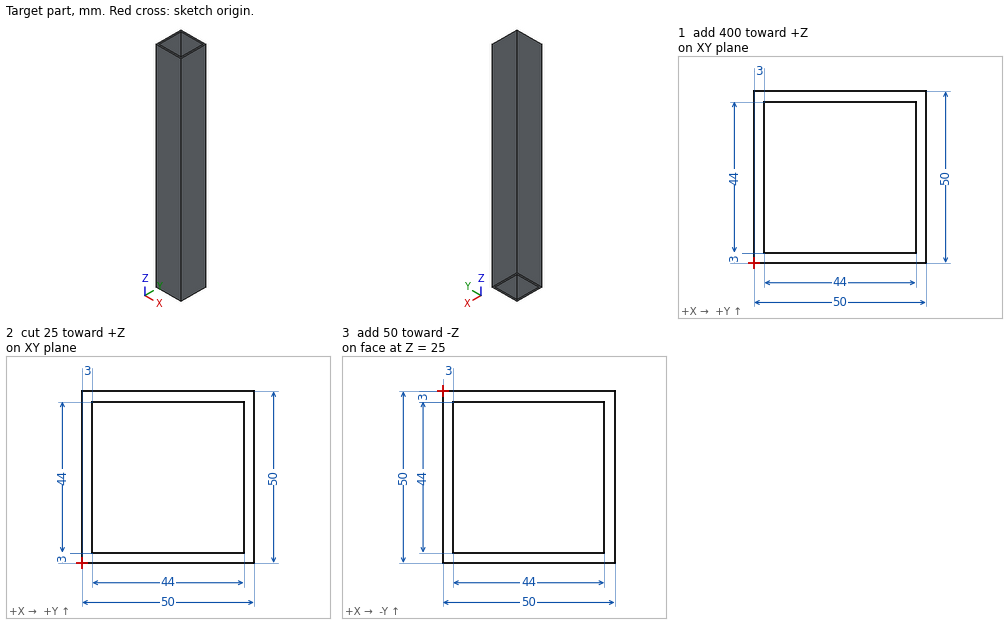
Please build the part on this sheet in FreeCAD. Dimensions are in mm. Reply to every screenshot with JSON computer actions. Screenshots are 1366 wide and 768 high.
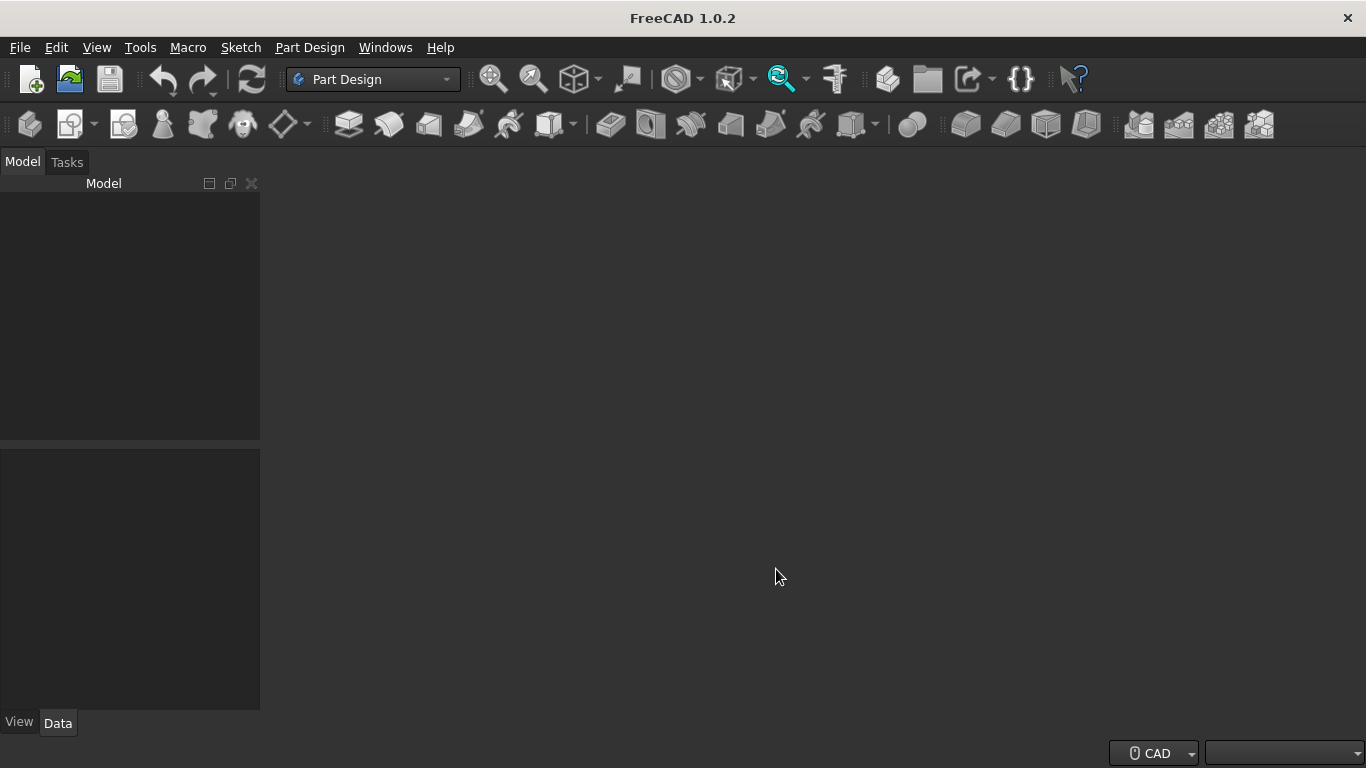
{"action": "left_click", "coordinate": [30, 80]}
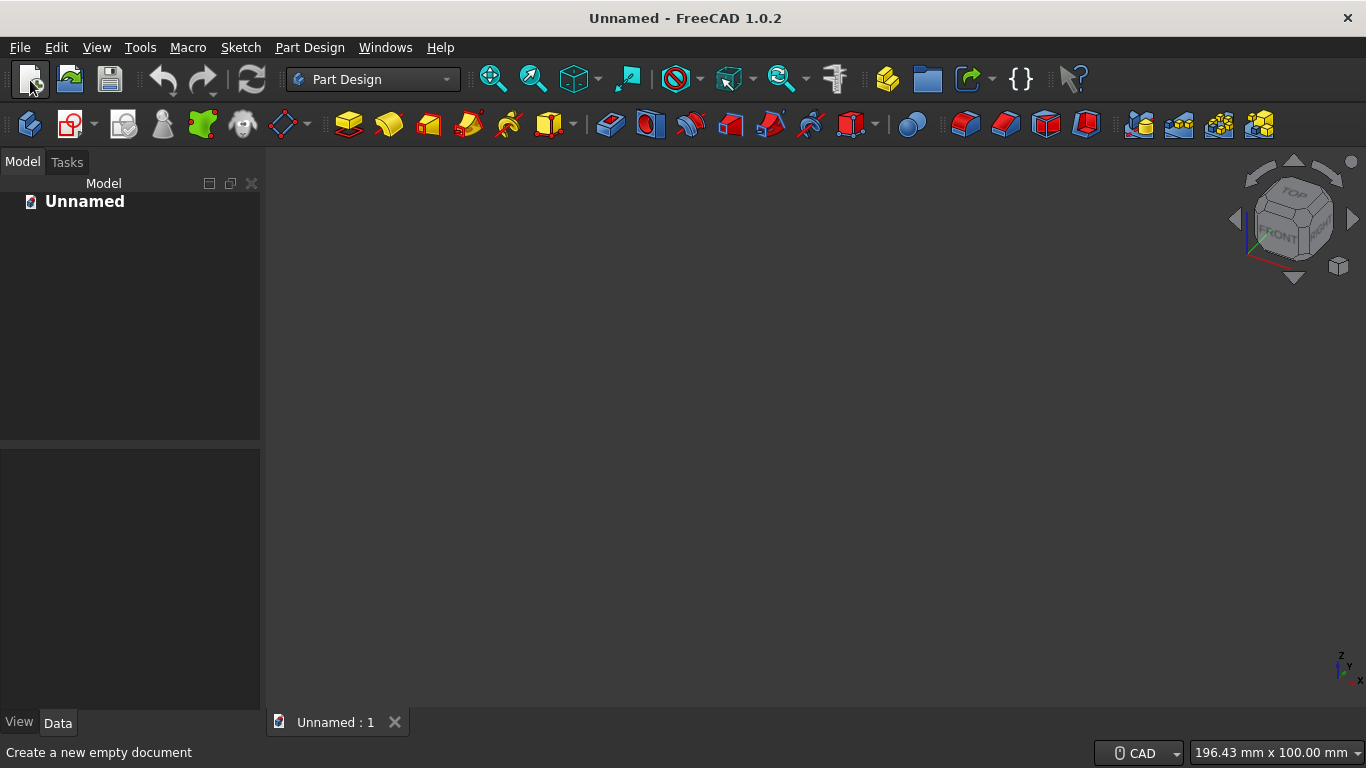
{"action": "left_click", "coordinate": [70, 124]}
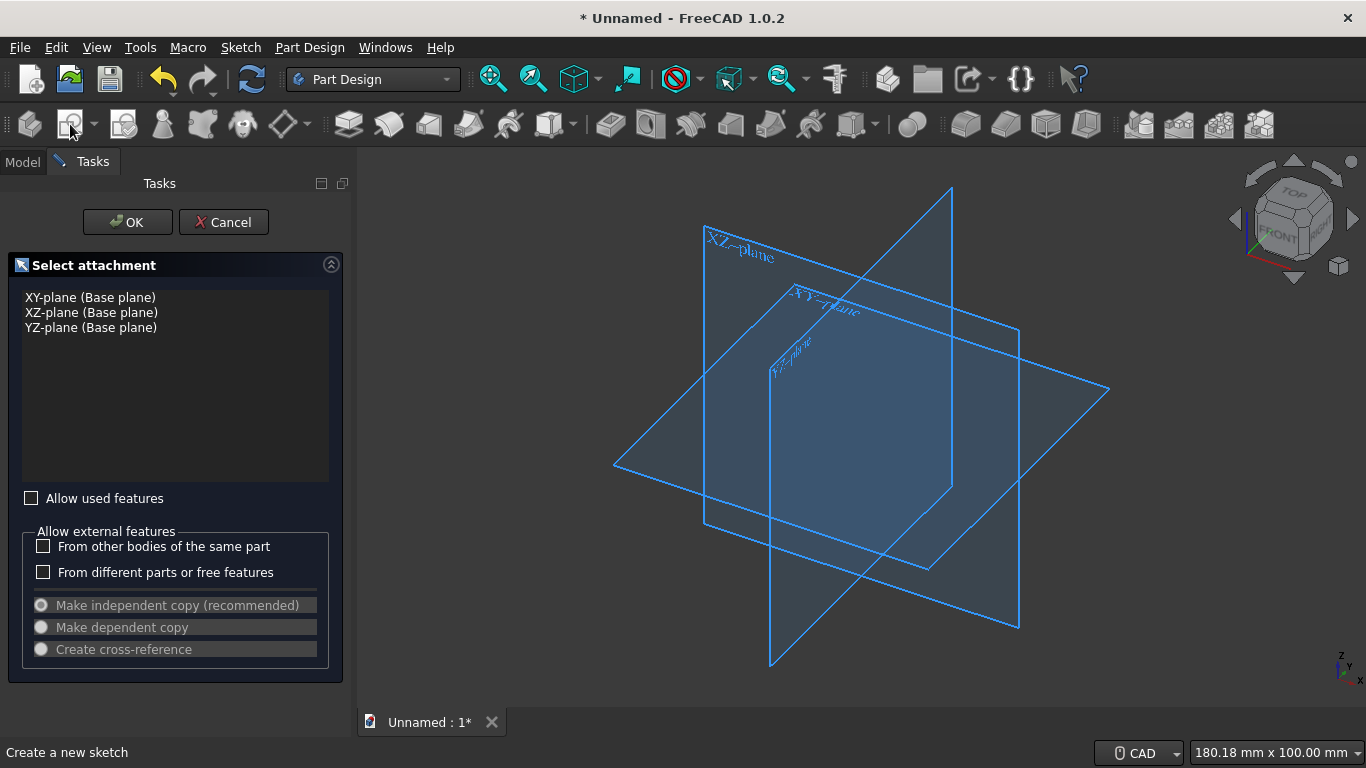
{"action": "left_click", "coordinate": [82, 298]}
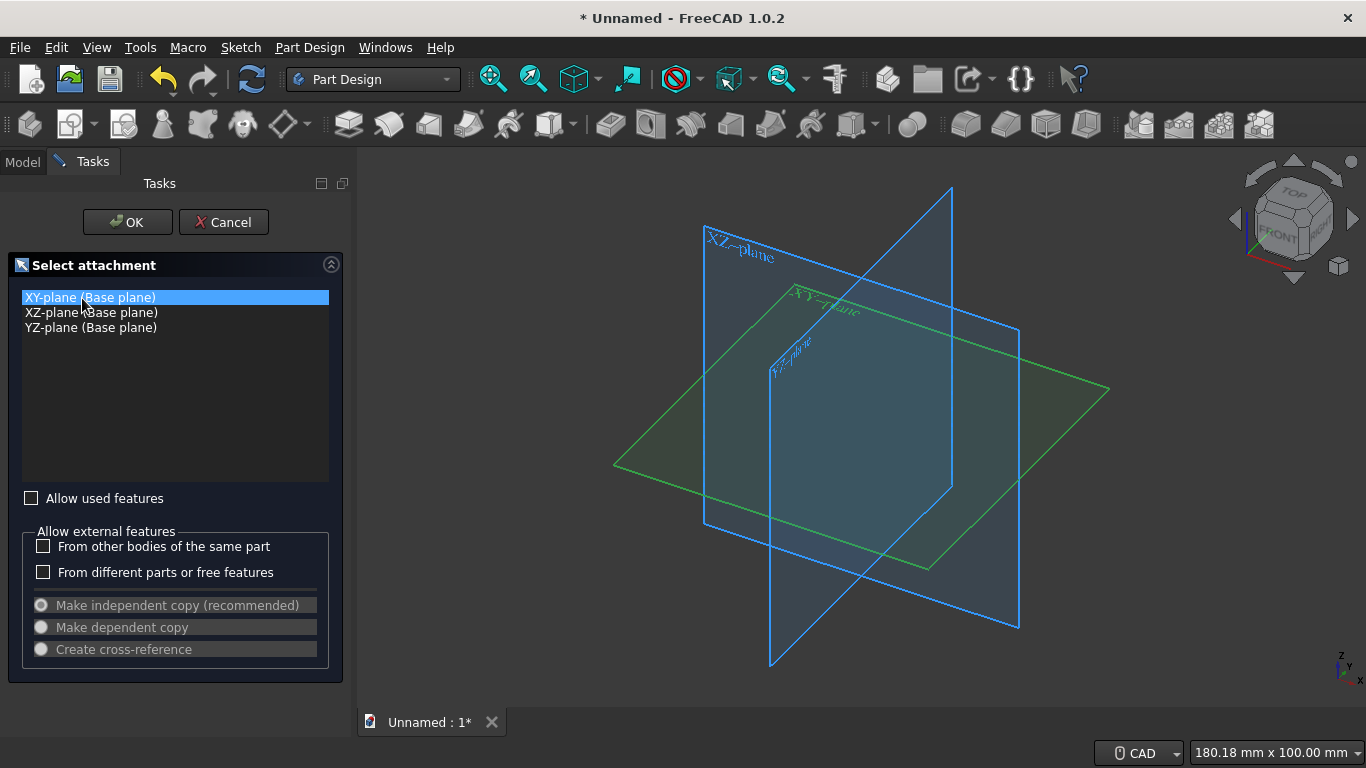
{"action": "left_click", "coordinate": [128, 222]}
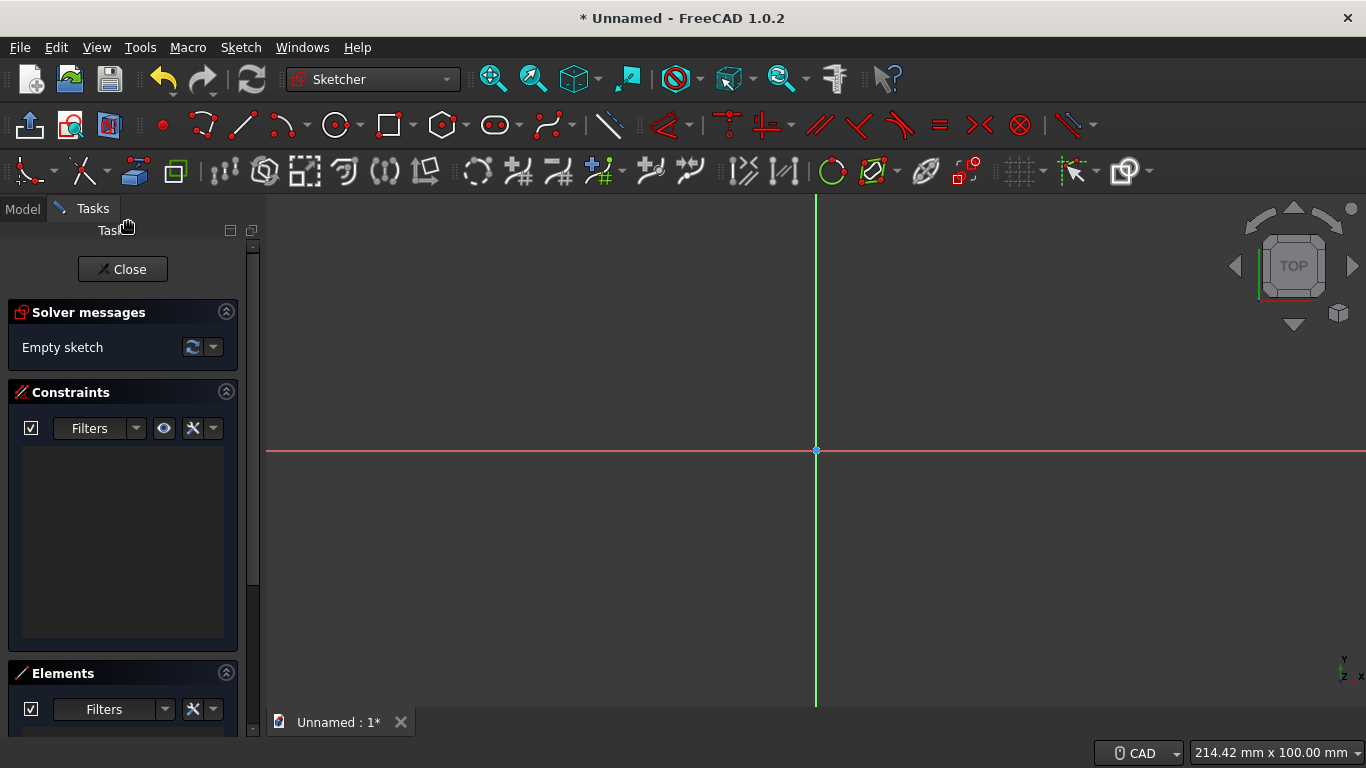
{"action": "scroll", "coordinate": [294, 679], "scroll_direction": "down", "scroll_amount": 1}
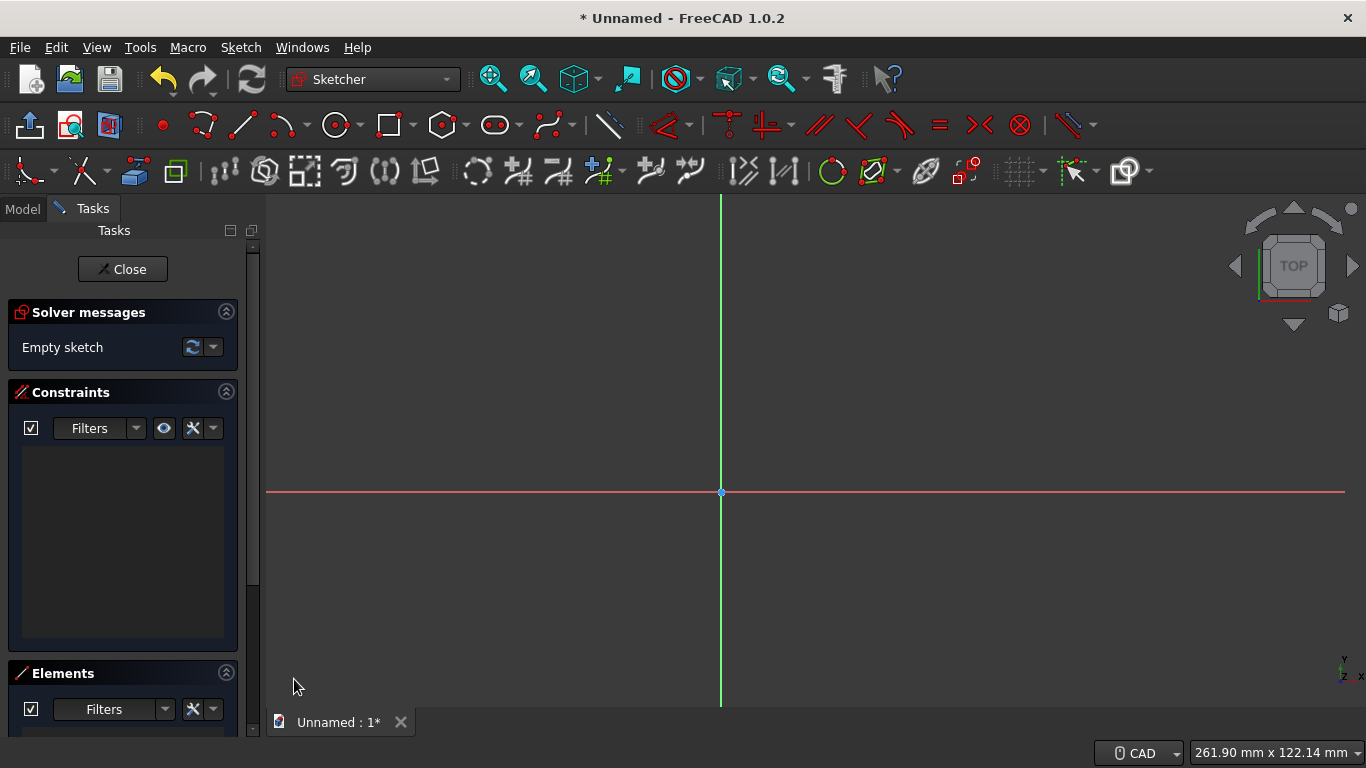
{"action": "scroll", "coordinate": [987, 258], "scroll_direction": "up", "scroll_amount": 2}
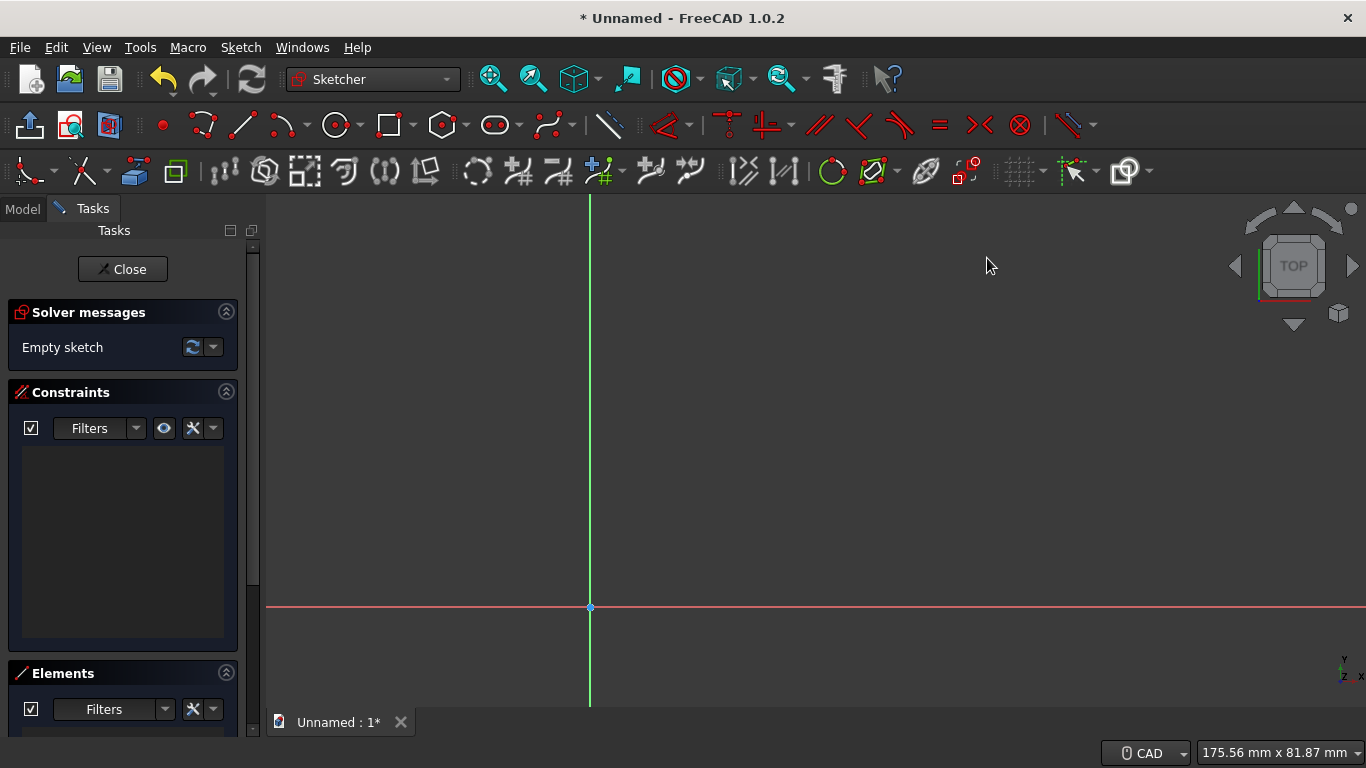
{"action": "left_click", "coordinate": [390, 126]}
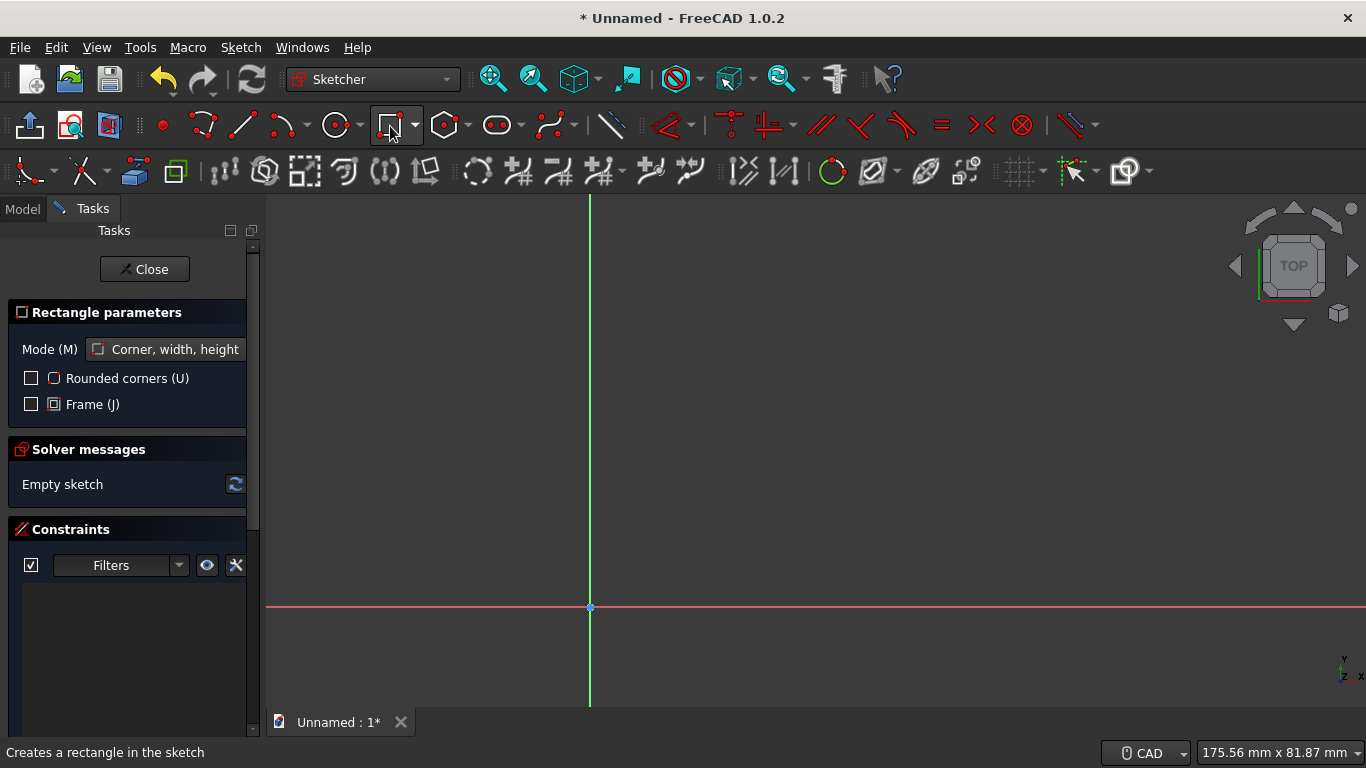
{"action": "left_click", "coordinate": [590, 607]}
{"action": "left_click", "coordinate": [904, 294]}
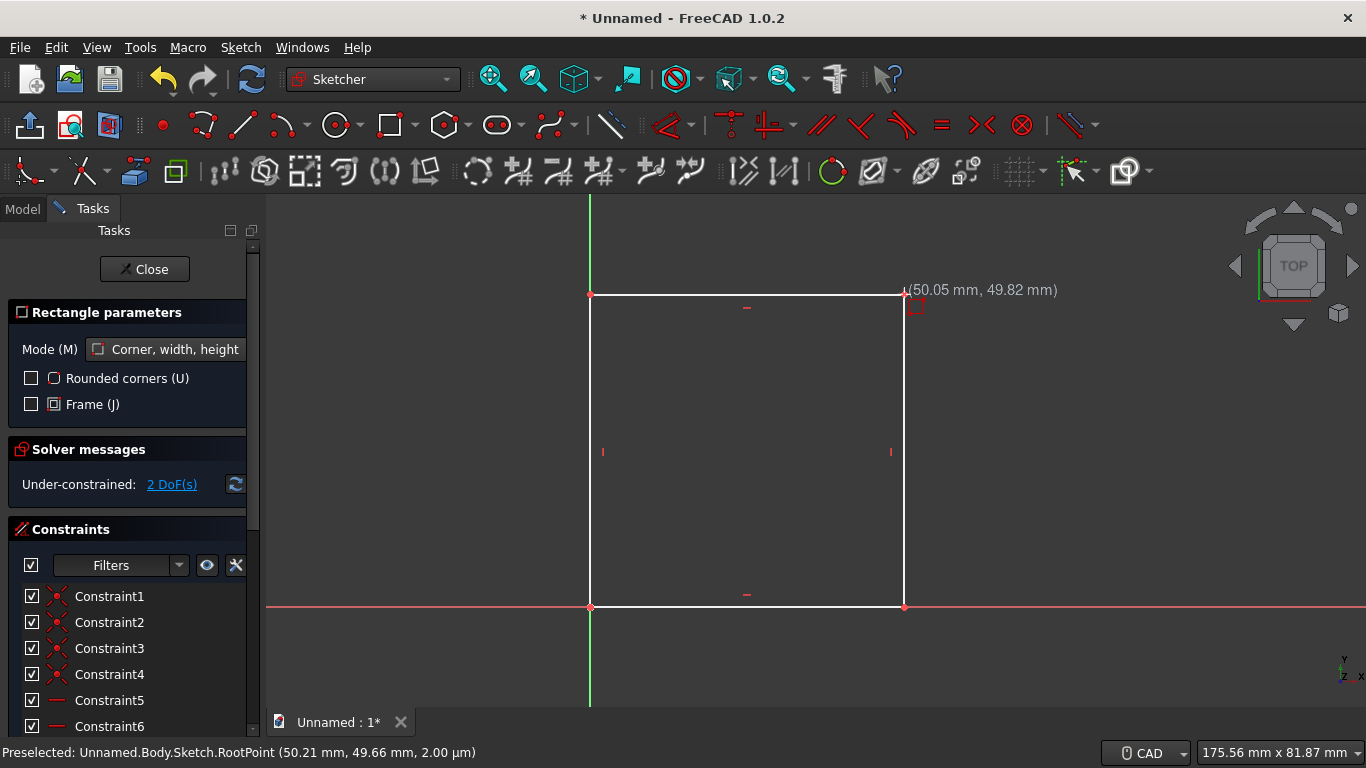
{"action": "left_click", "coordinate": [609, 313]}
{"action": "left_click", "coordinate": [885, 588]}
{"action": "key", "text": "Escape"}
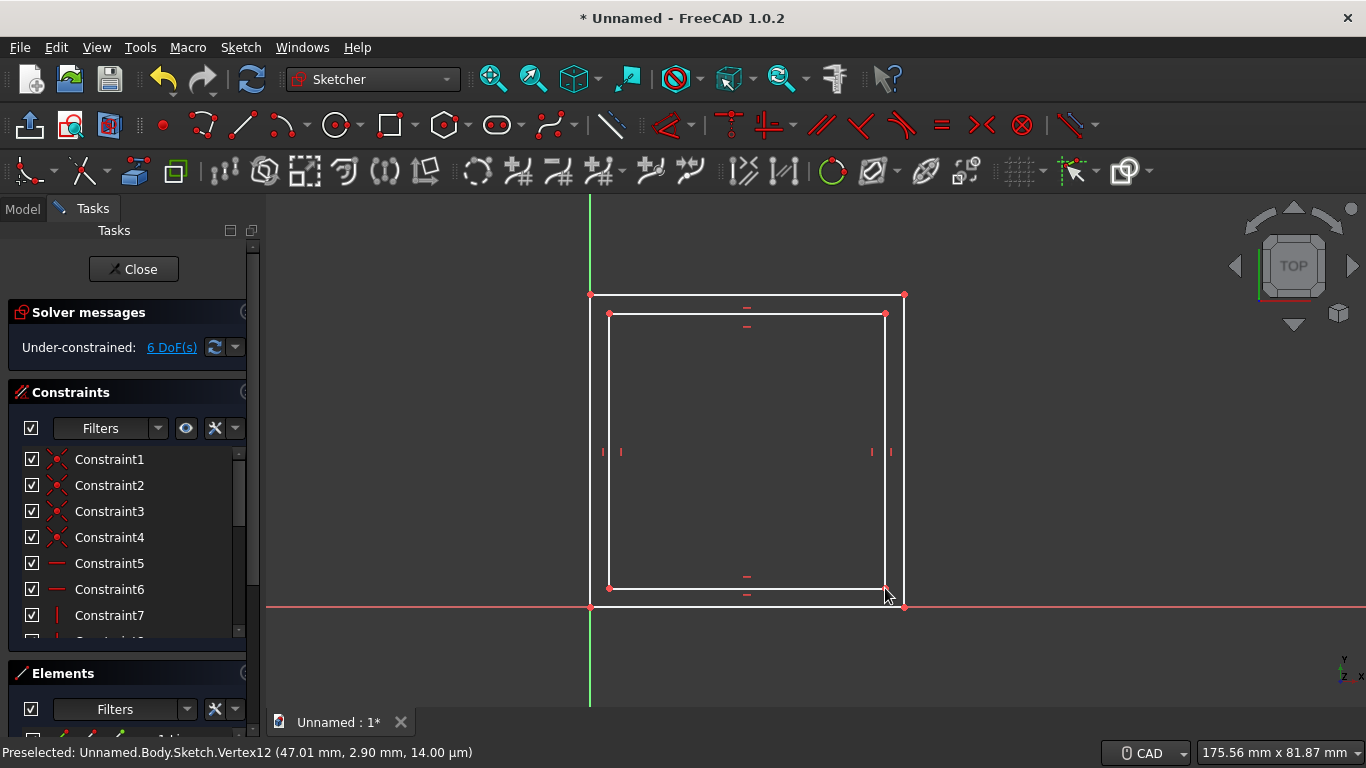
{"action": "left_click", "coordinate": [666, 126]}